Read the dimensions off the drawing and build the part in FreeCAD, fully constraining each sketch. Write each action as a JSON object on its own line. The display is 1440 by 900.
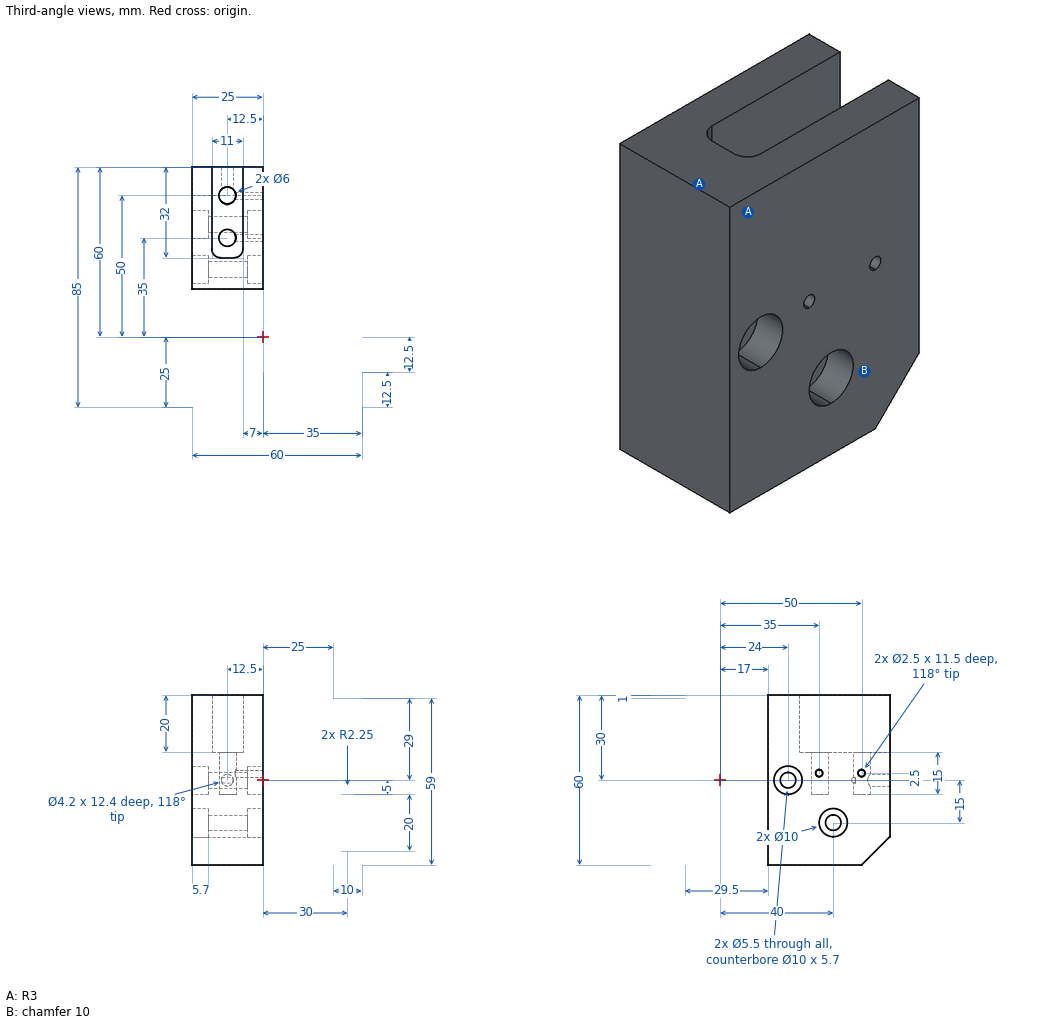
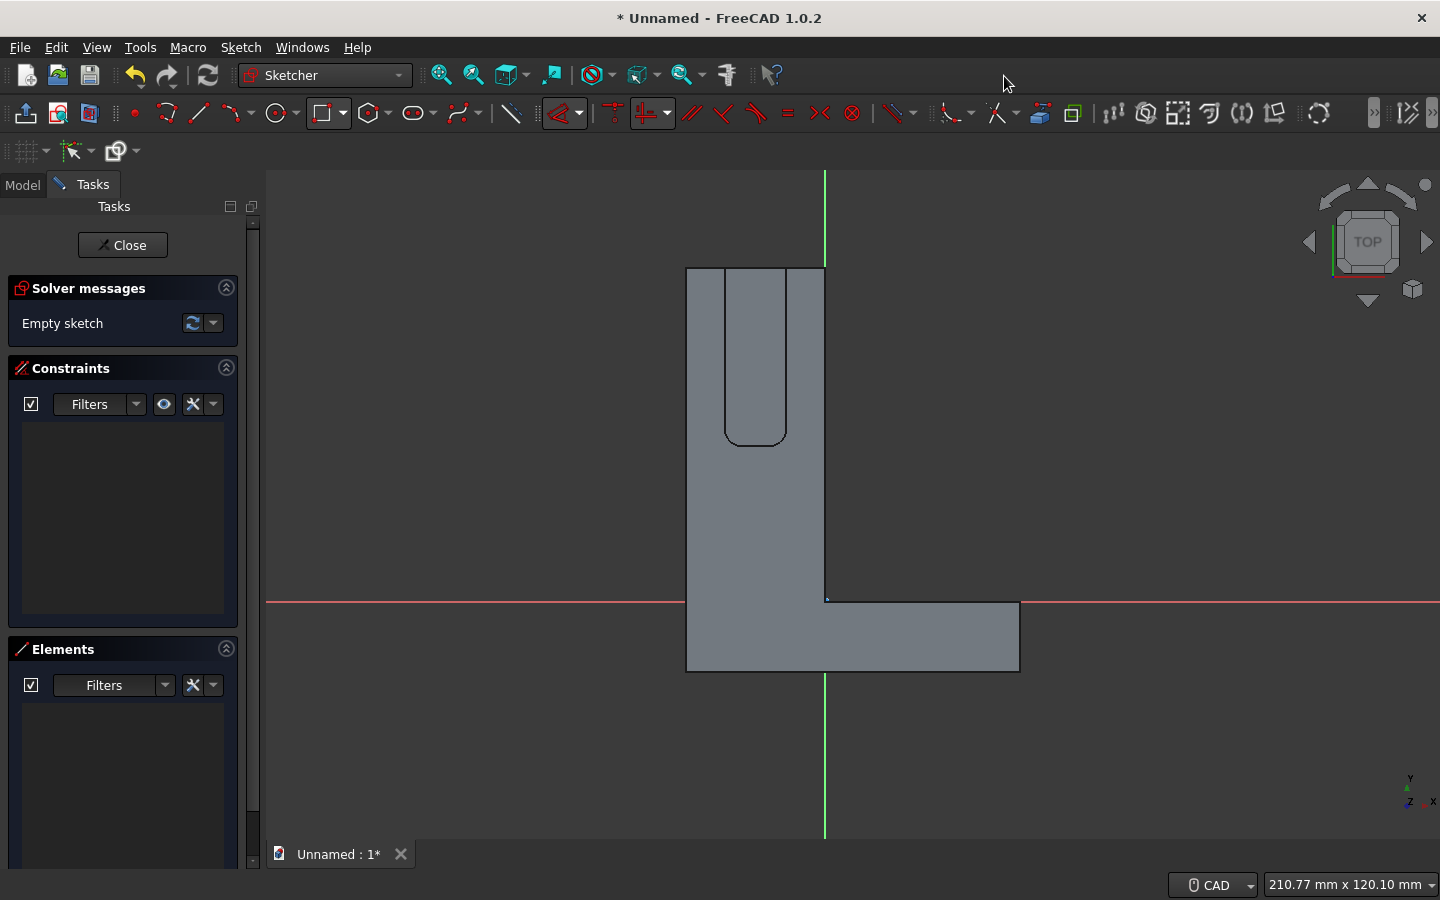
{"action": "left_click", "coordinate": [90, 114]}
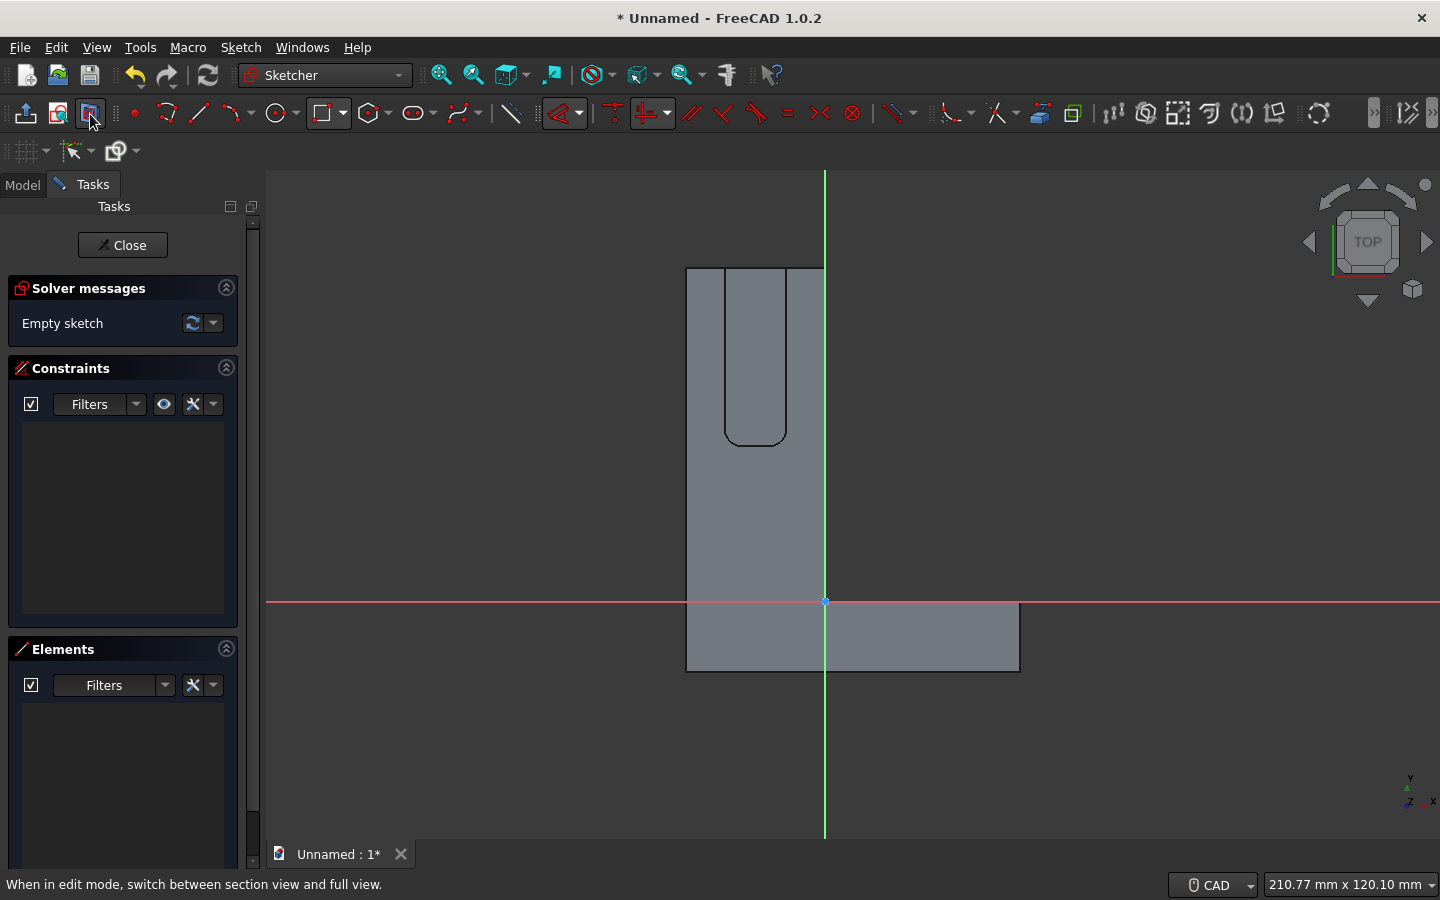
{"action": "scroll", "coordinate": [746, 320], "scroll_direction": "up", "scroll_amount": 7}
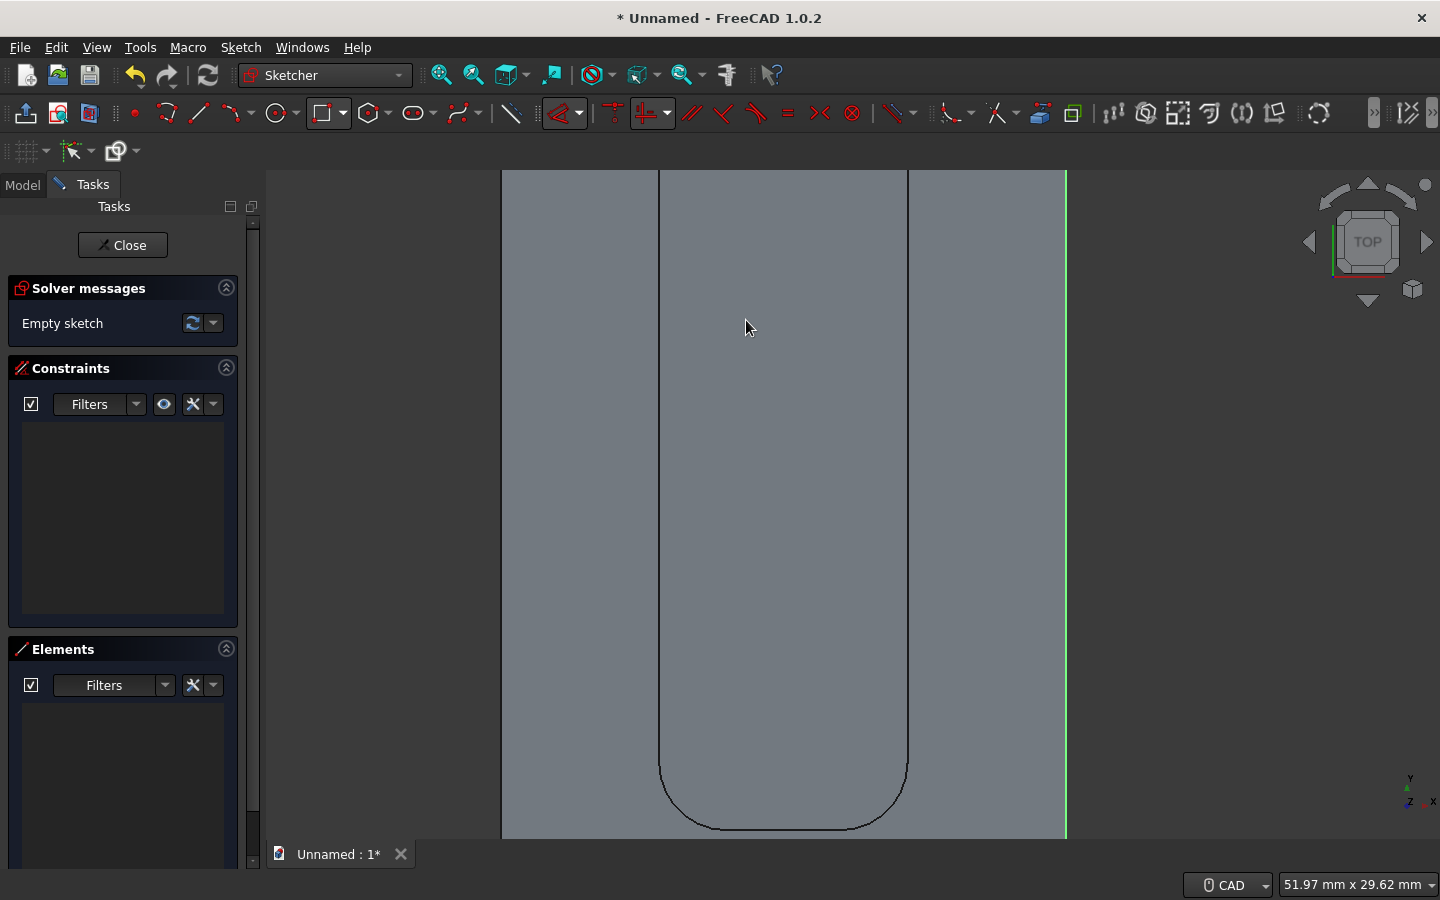
{"action": "left_click", "coordinate": [276, 114]}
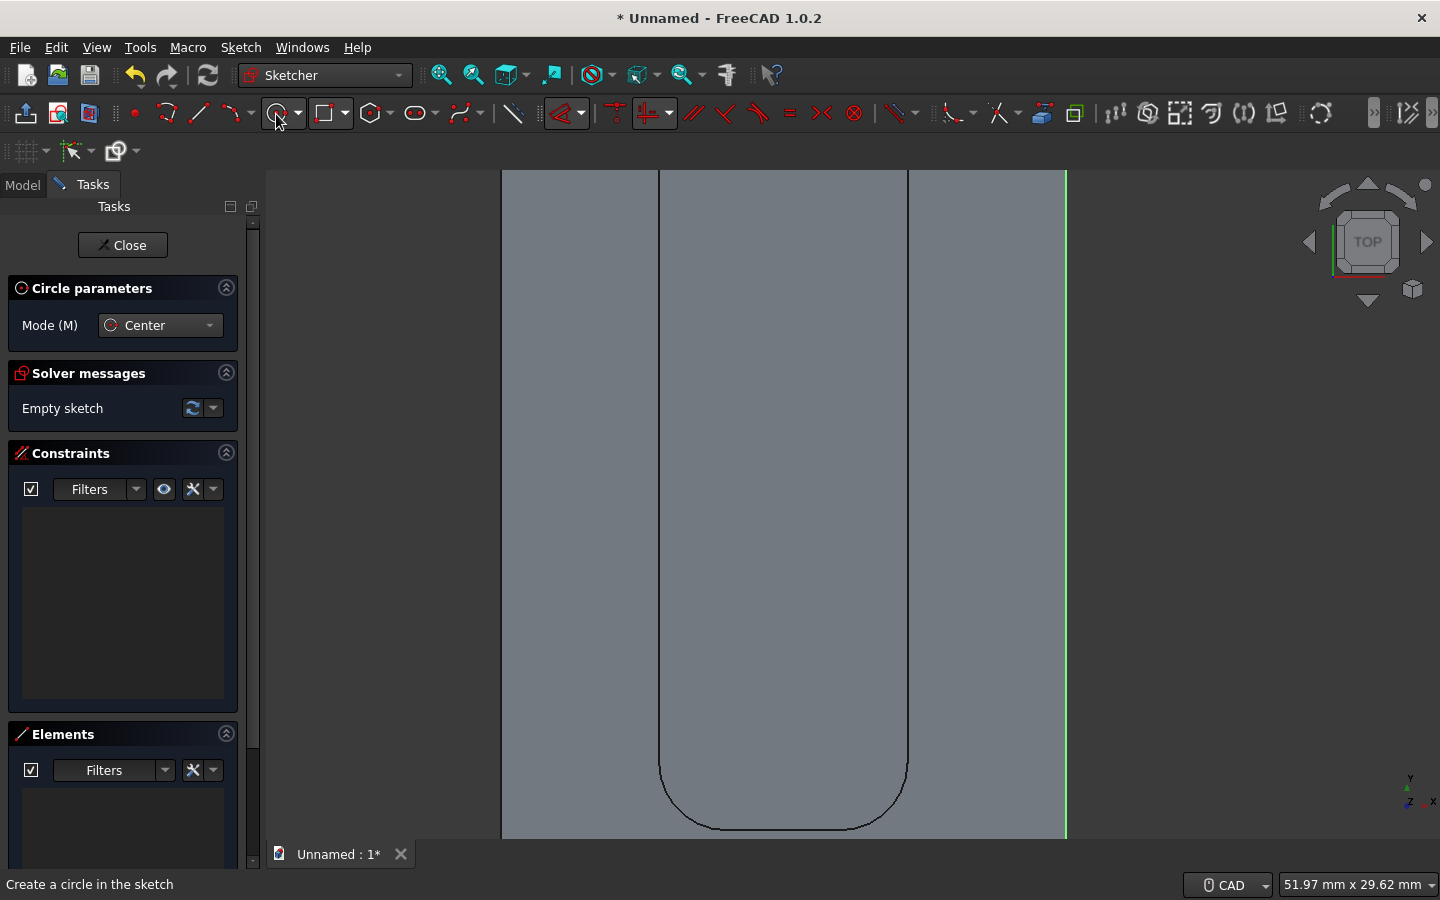
{"action": "left_click", "coordinate": [783, 333]}
{"action": "mouse_move", "coordinate": [831, 285]}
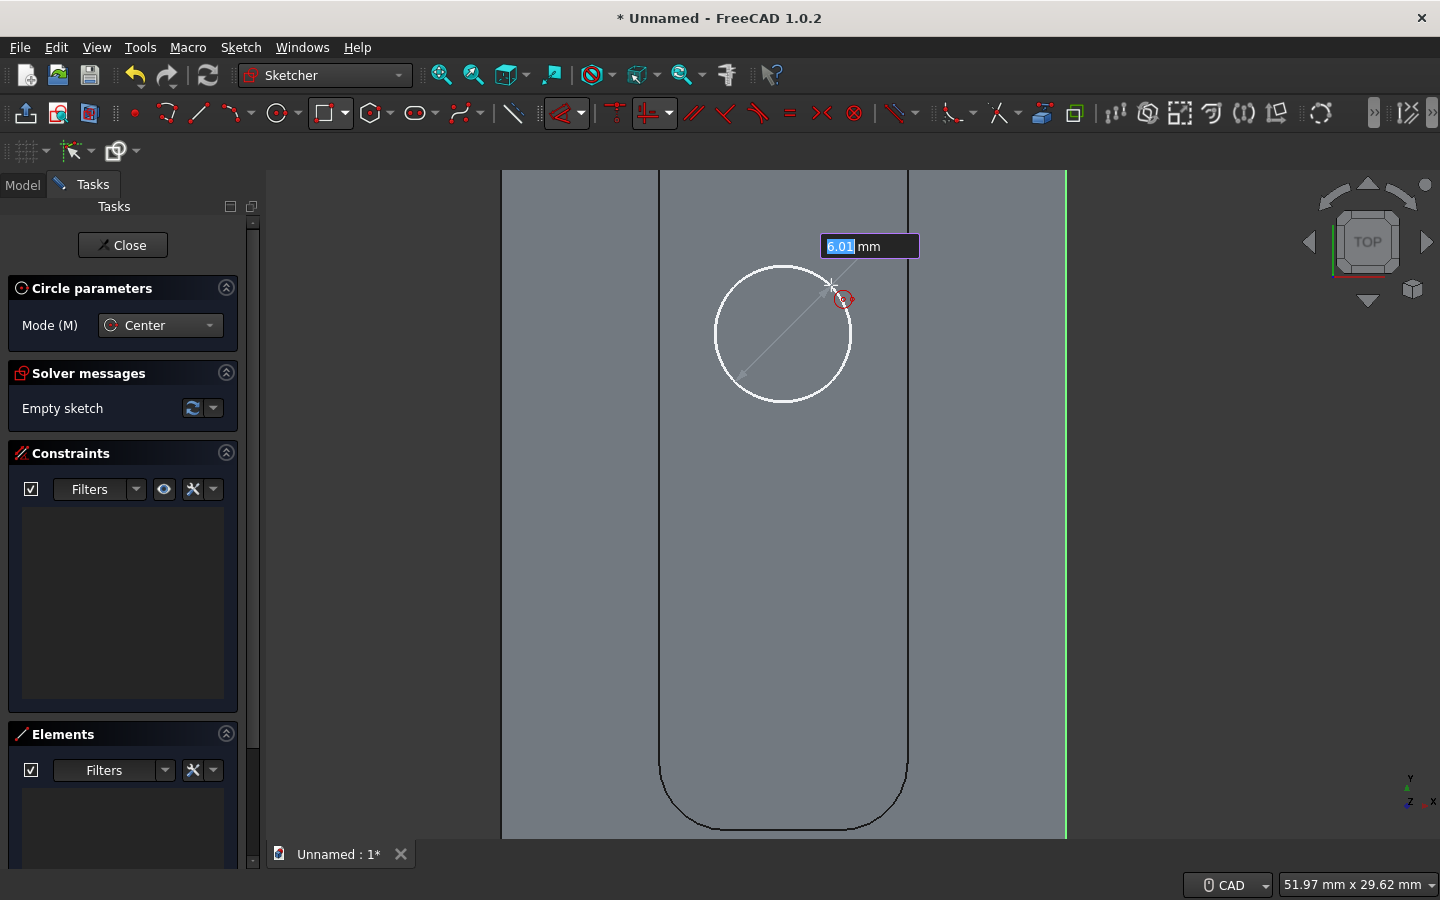
{"action": "type", "text": "6"}
{"action": "key", "text": "Return"}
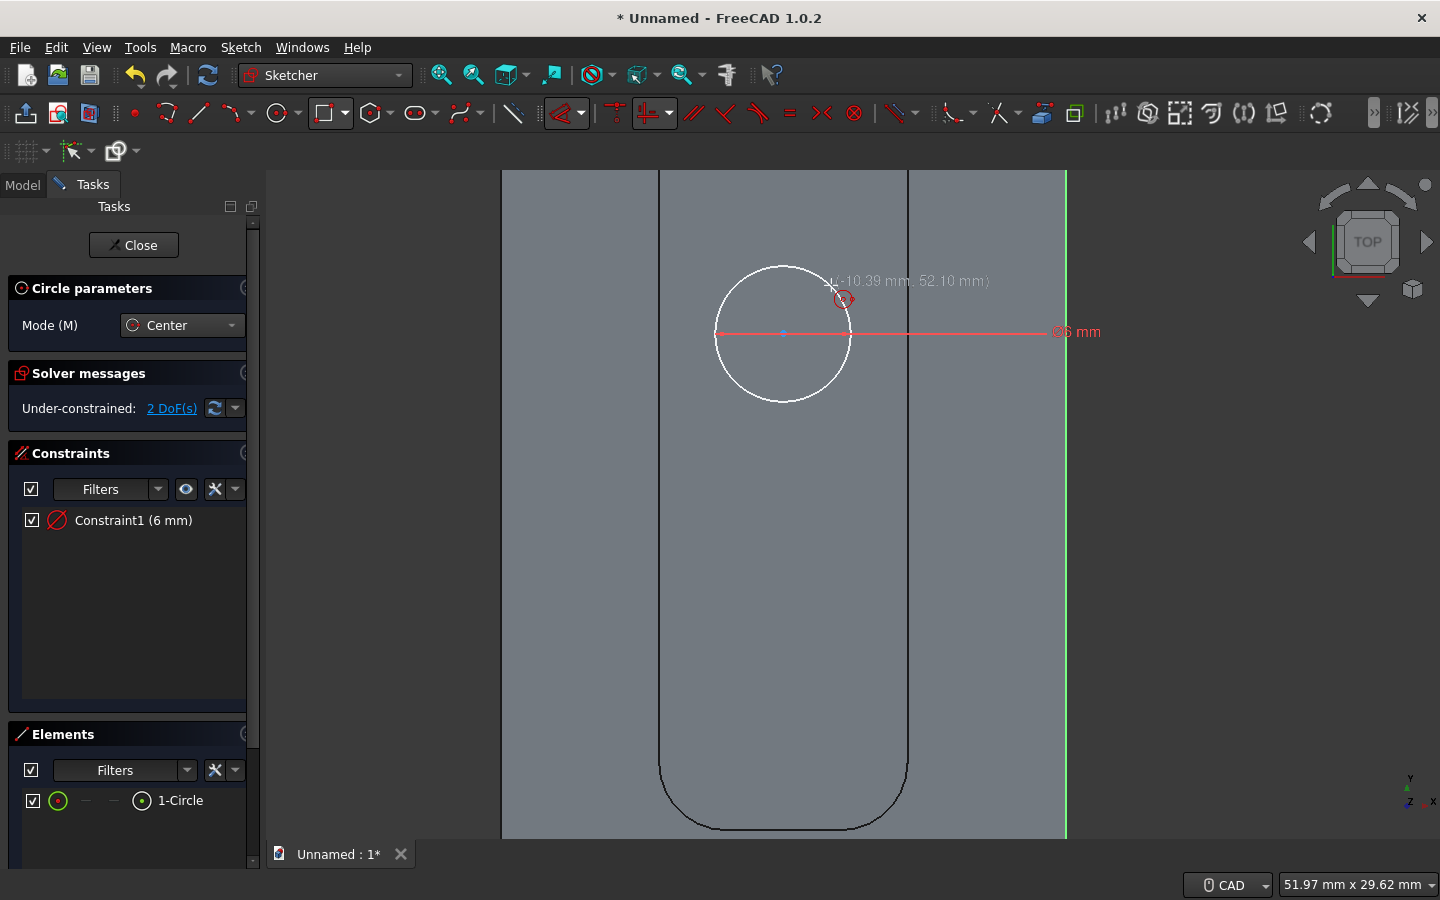
{"action": "left_click", "coordinate": [783, 672]}
{"action": "mouse_move", "coordinate": [831, 624]}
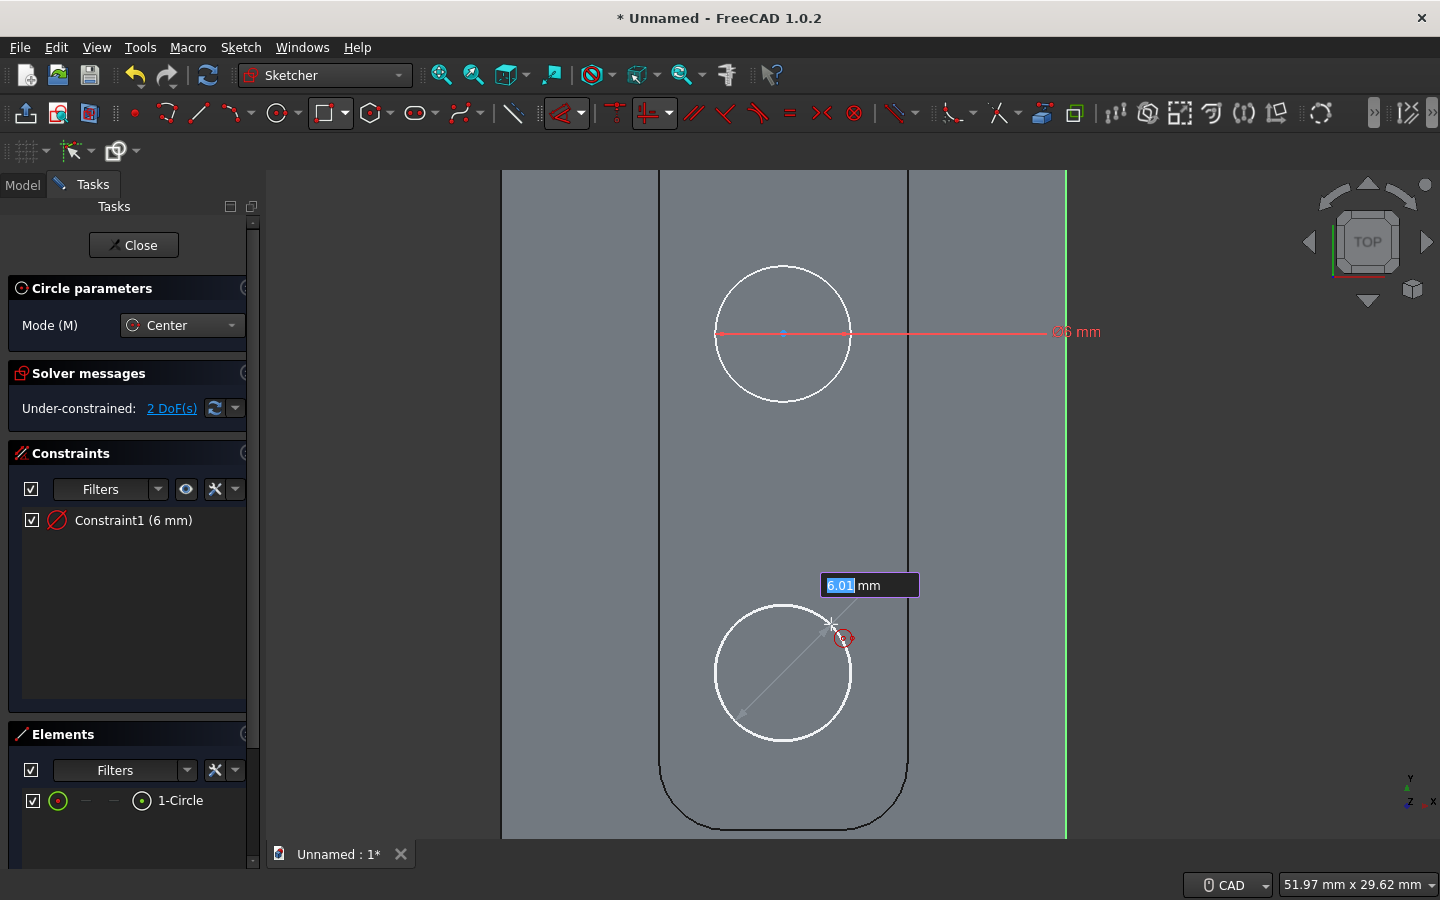
{"action": "type", "text": "6"}
{"action": "key", "text": "Return"}
{"action": "key", "text": "Escape"}